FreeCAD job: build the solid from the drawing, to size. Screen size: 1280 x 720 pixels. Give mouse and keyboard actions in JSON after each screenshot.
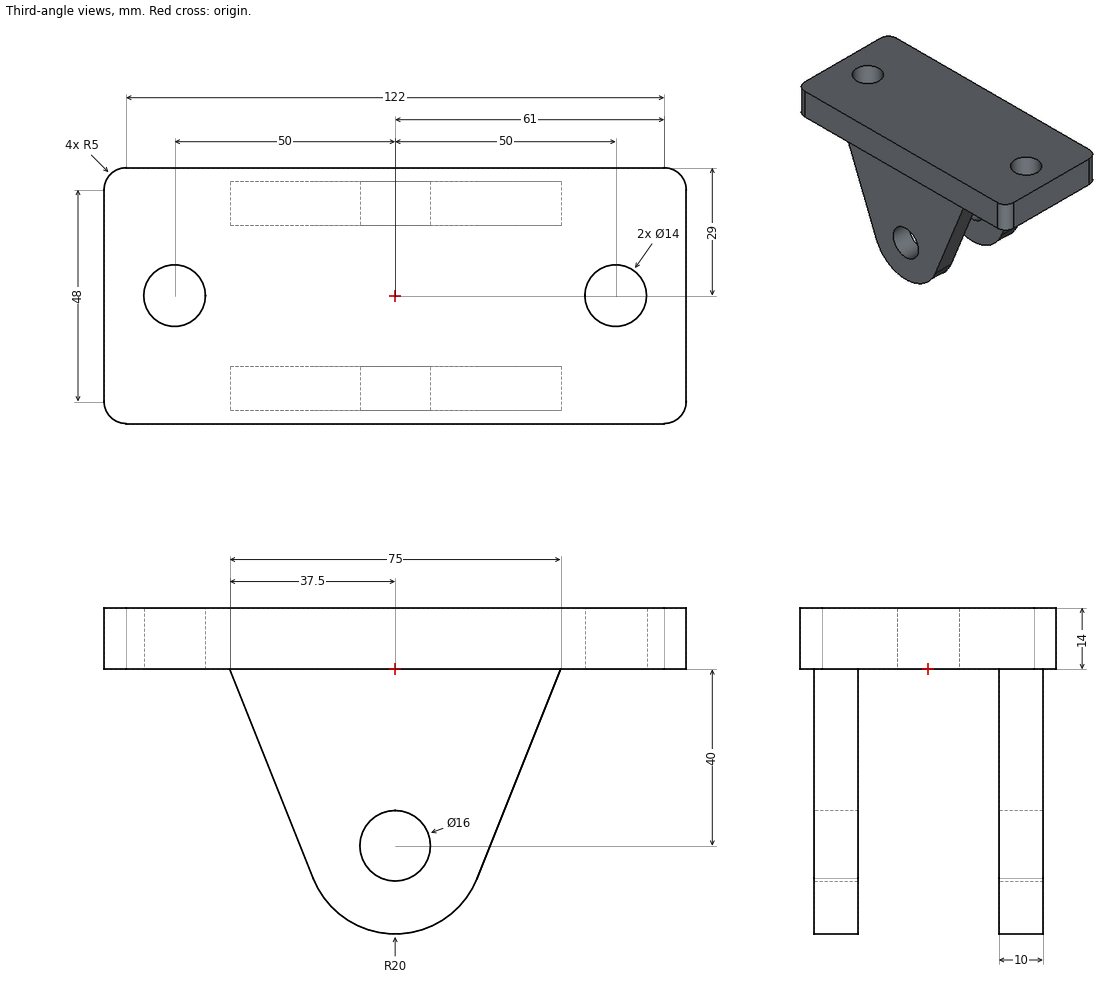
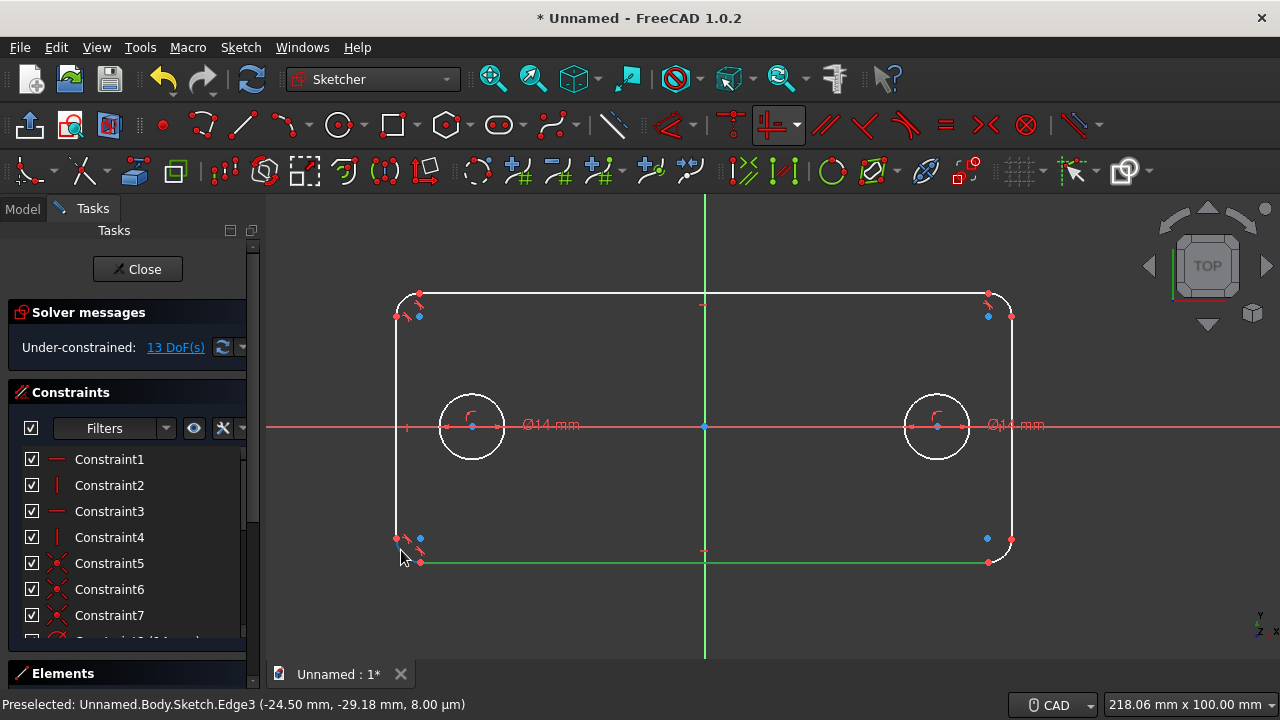
{"action": "scroll", "coordinate": [999, 560], "scroll_direction": "up", "scroll_amount": 2}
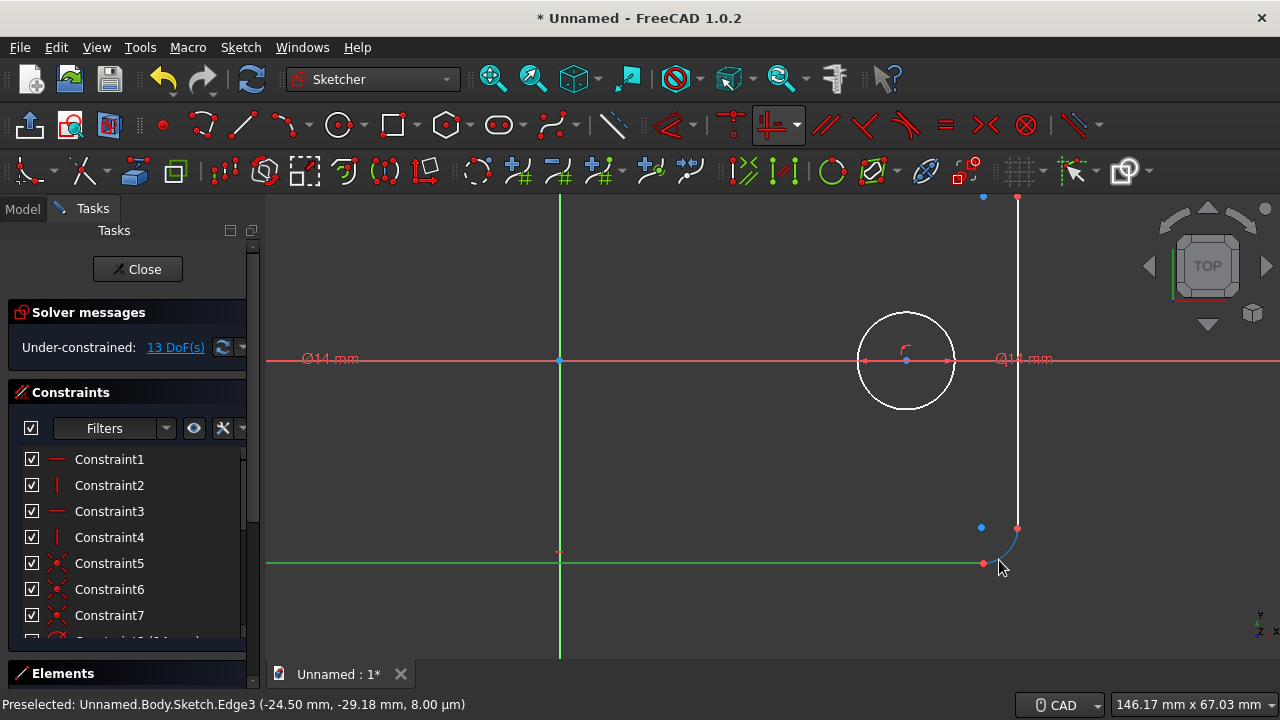
{"action": "left_click", "coordinate": [999, 559]}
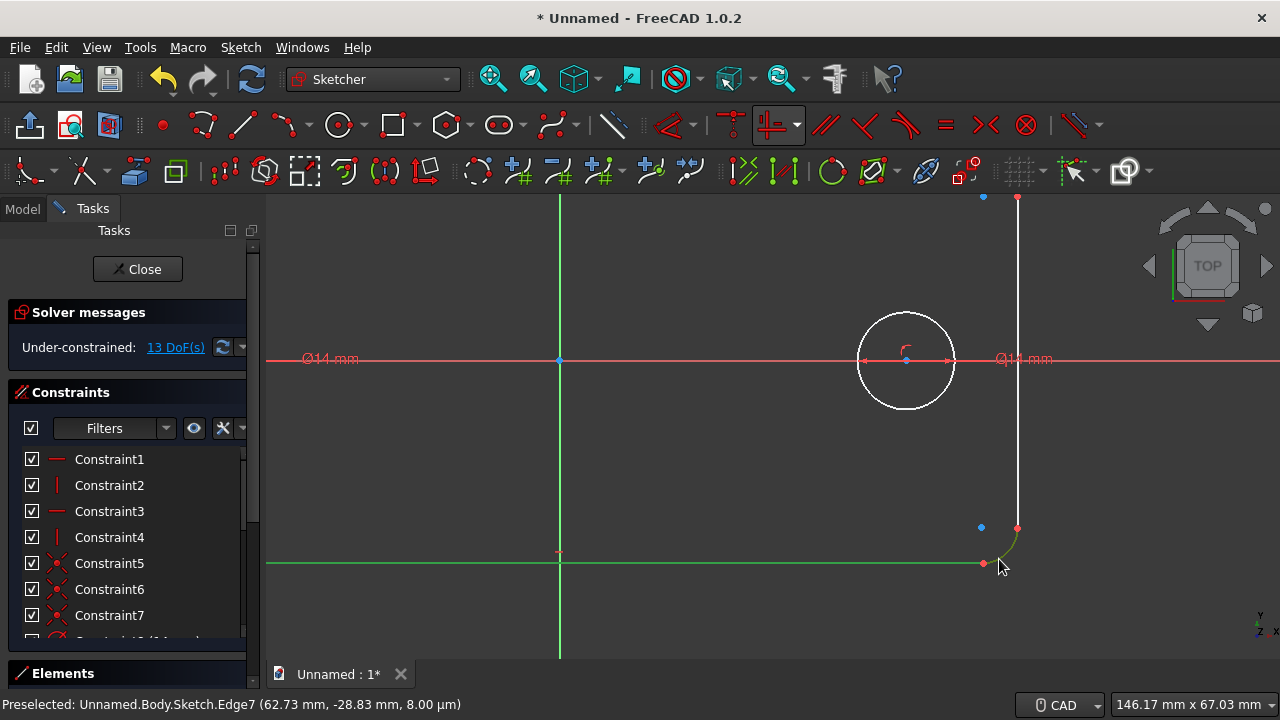
{"action": "left_click", "coordinate": [906, 126]}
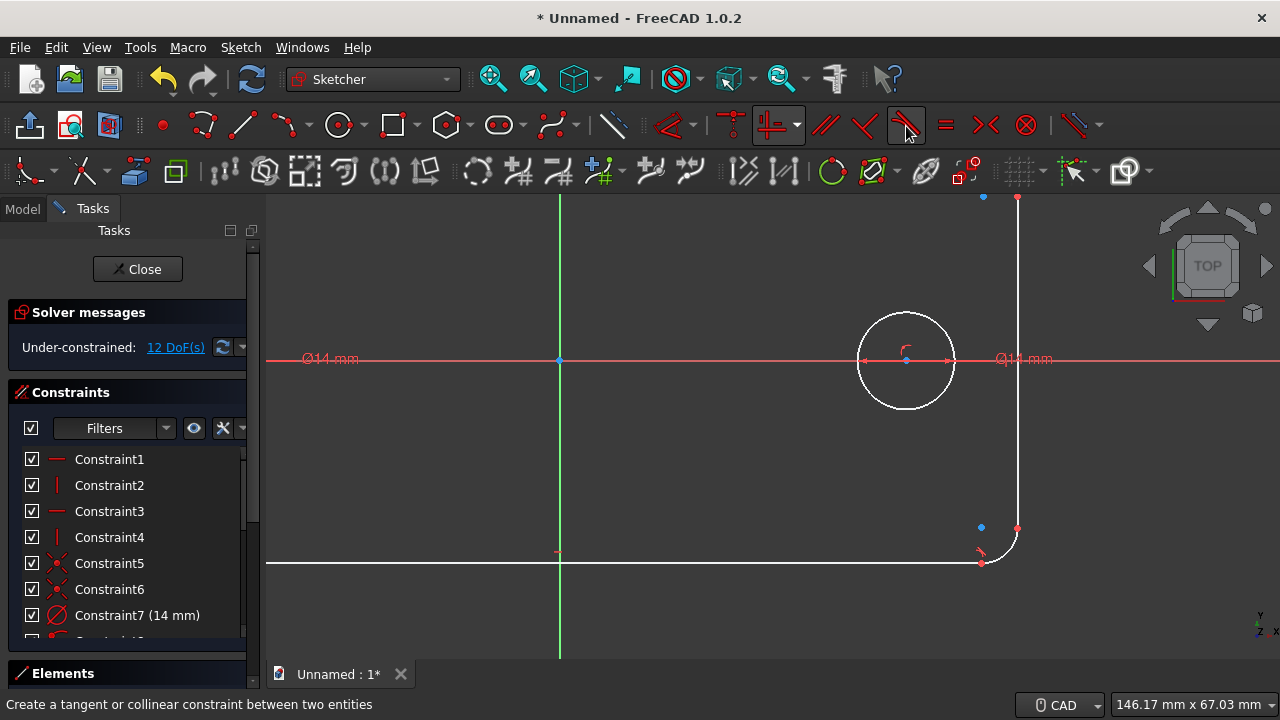
{"action": "left_click", "coordinate": [1018, 429]}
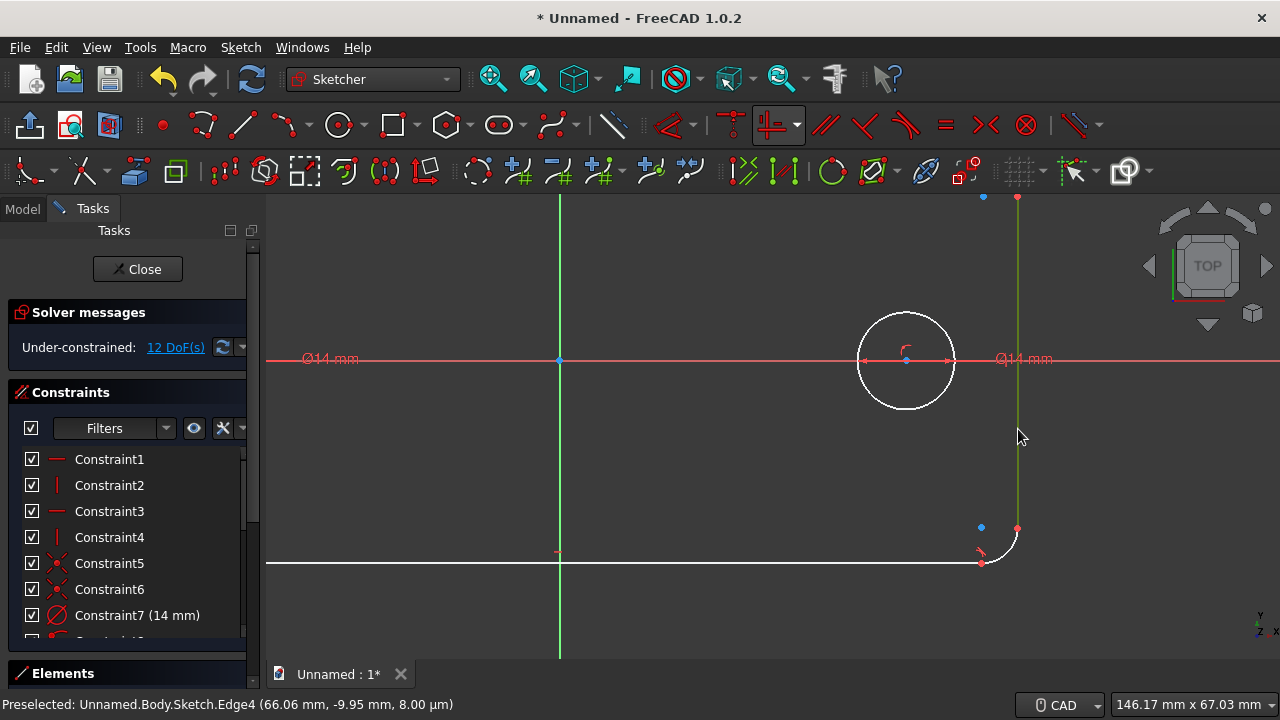
{"action": "left_click", "coordinate": [998, 560]}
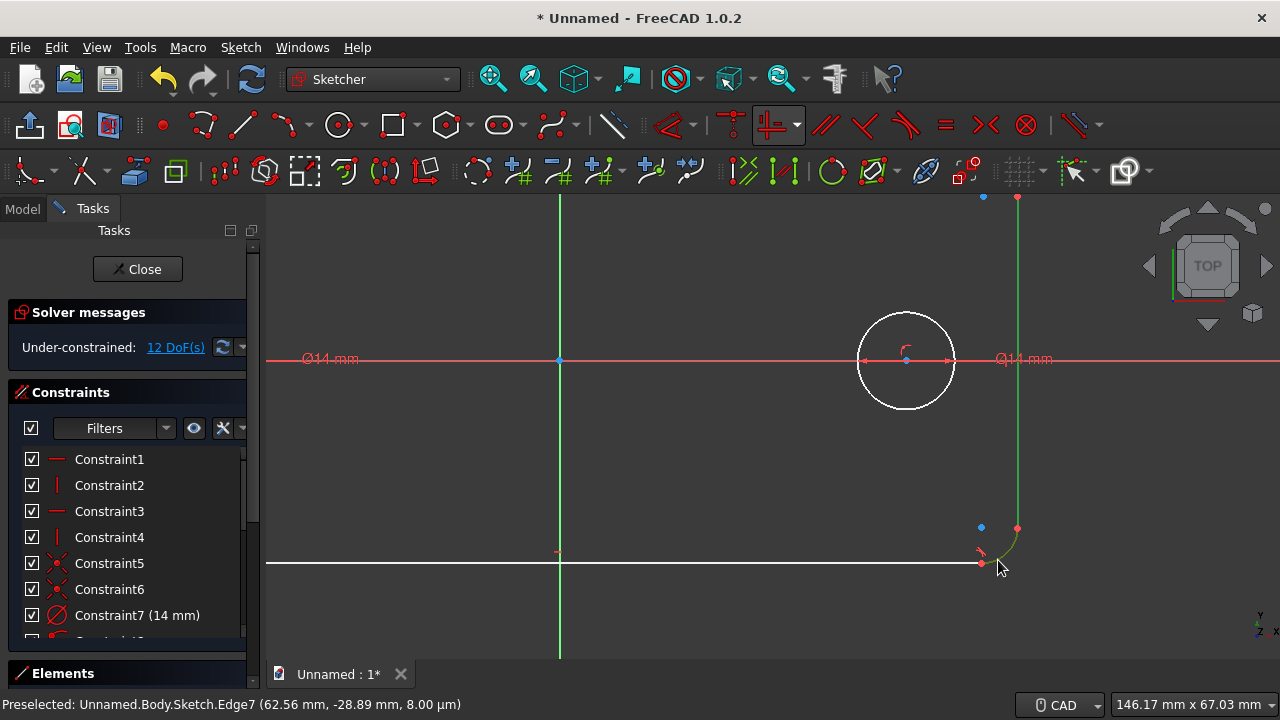
{"action": "left_click", "coordinate": [906, 126]}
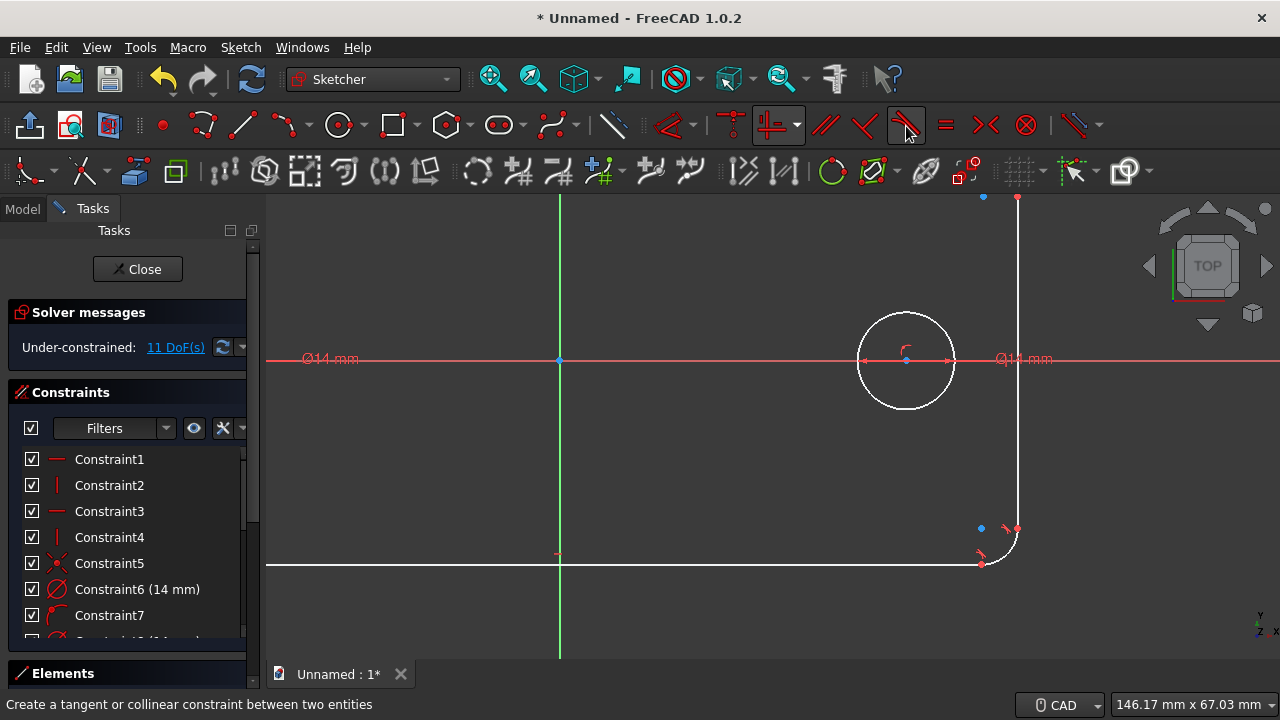
{"action": "left_click", "coordinate": [1018, 429]}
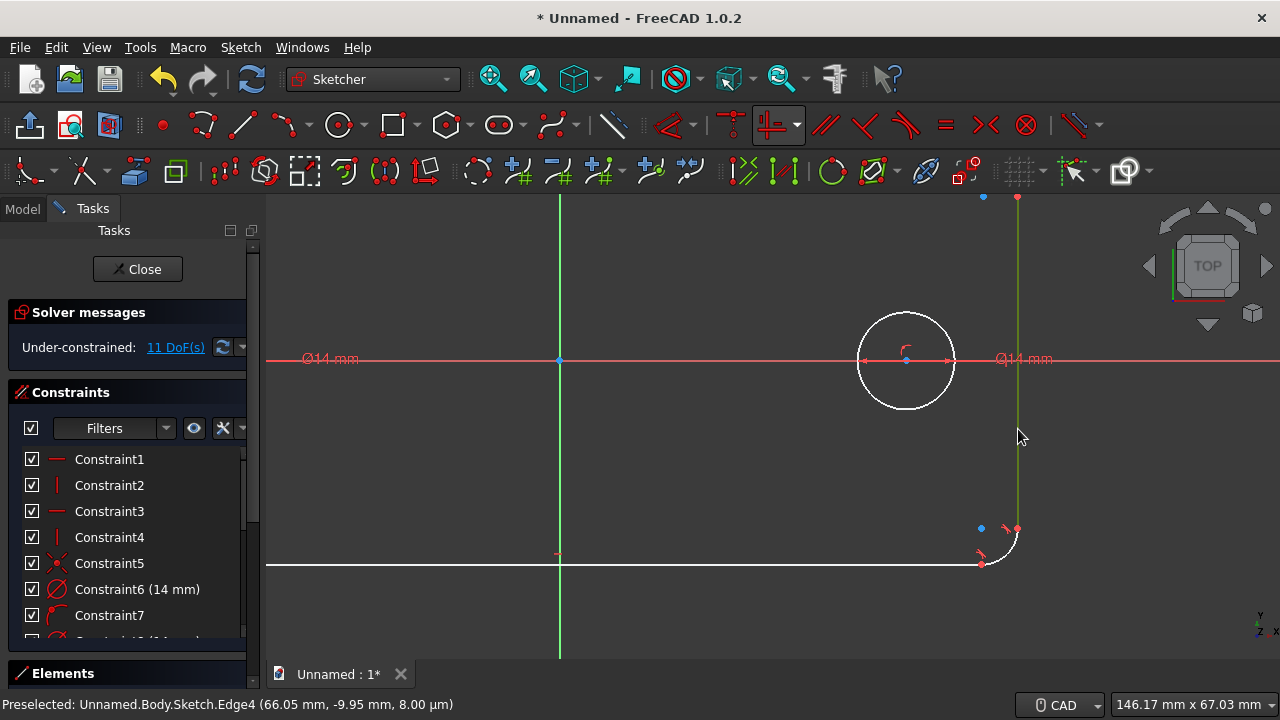
{"action": "scroll", "coordinate": [999, 560], "scroll_direction": "down", "scroll_amount": 2}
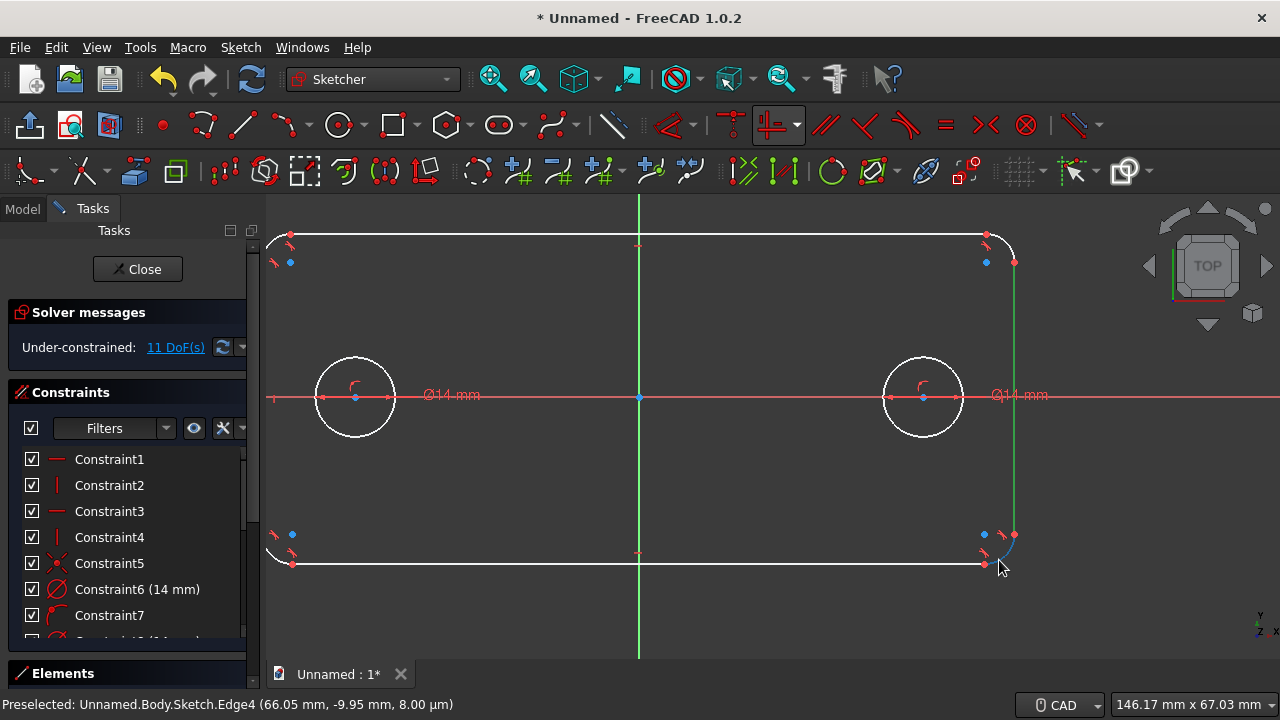
{"action": "scroll", "coordinate": [1009, 306], "scroll_direction": "up", "scroll_amount": 2}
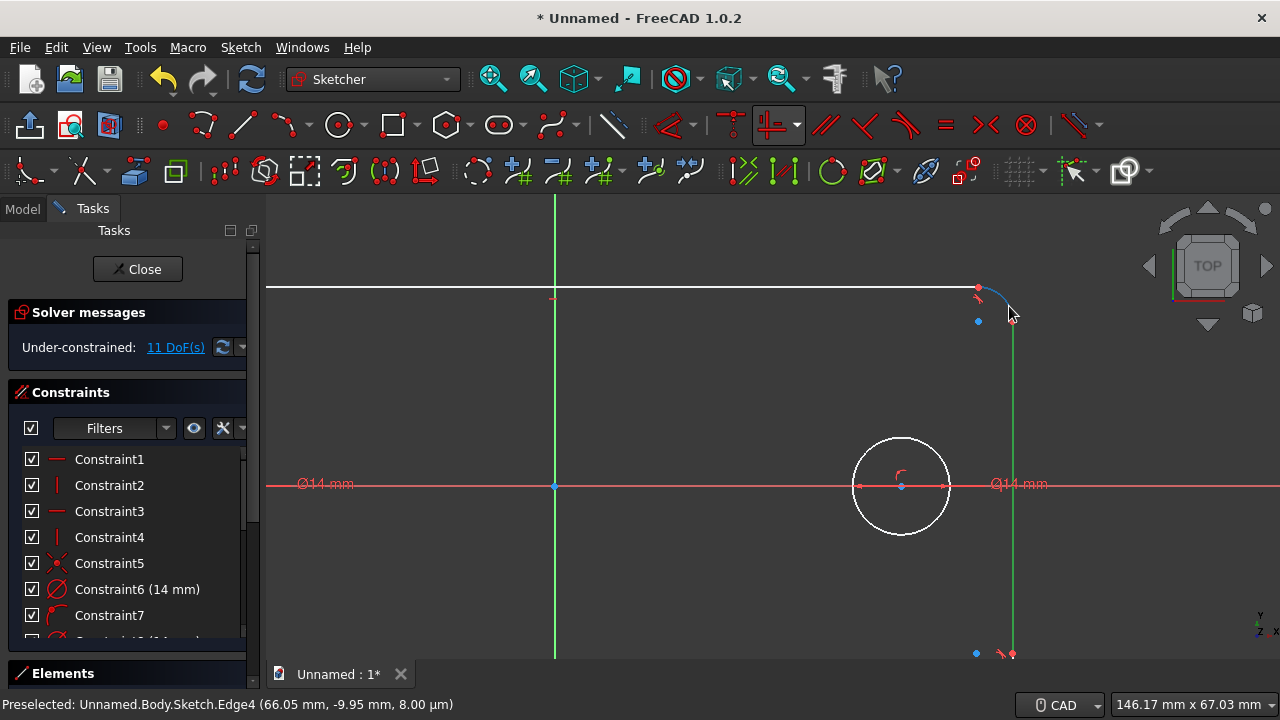
{"action": "left_click", "coordinate": [1009, 306]}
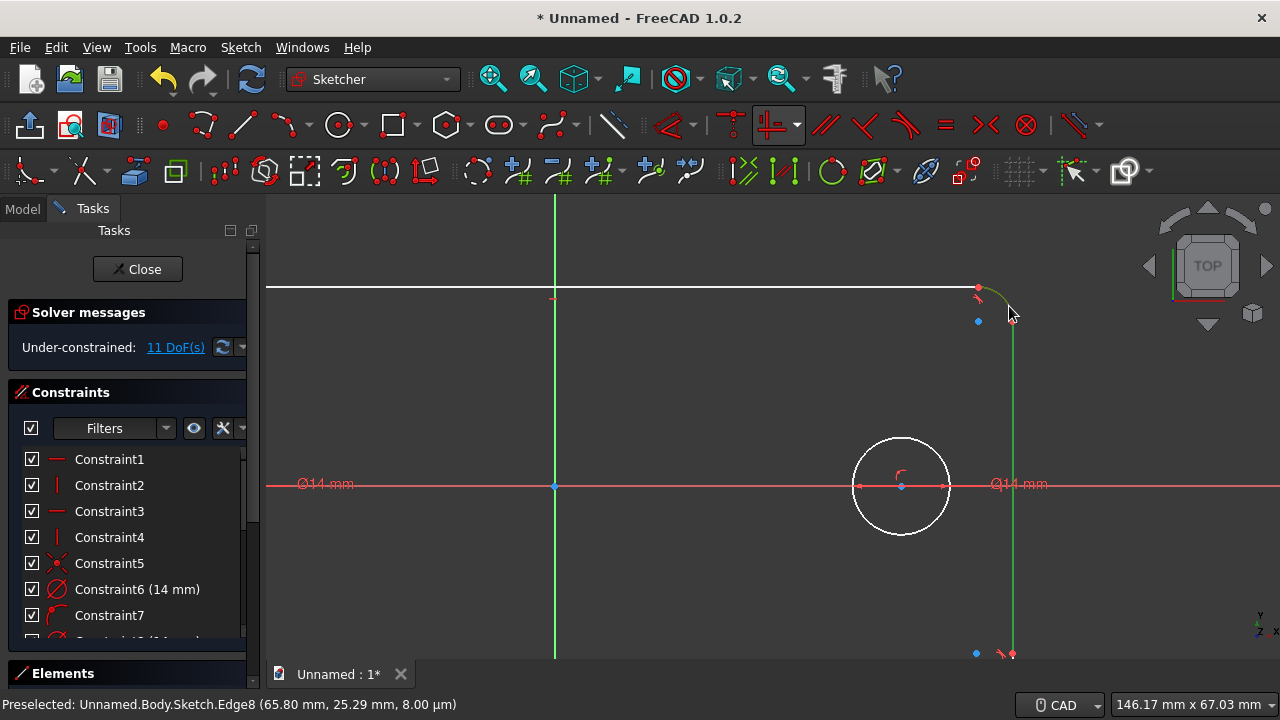
{"action": "left_click", "coordinate": [906, 126]}